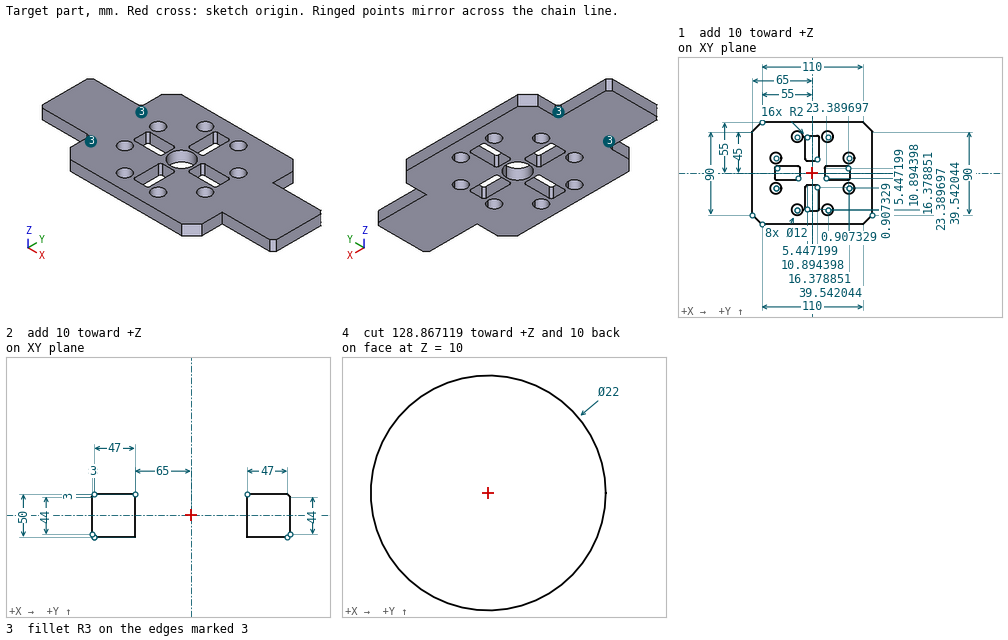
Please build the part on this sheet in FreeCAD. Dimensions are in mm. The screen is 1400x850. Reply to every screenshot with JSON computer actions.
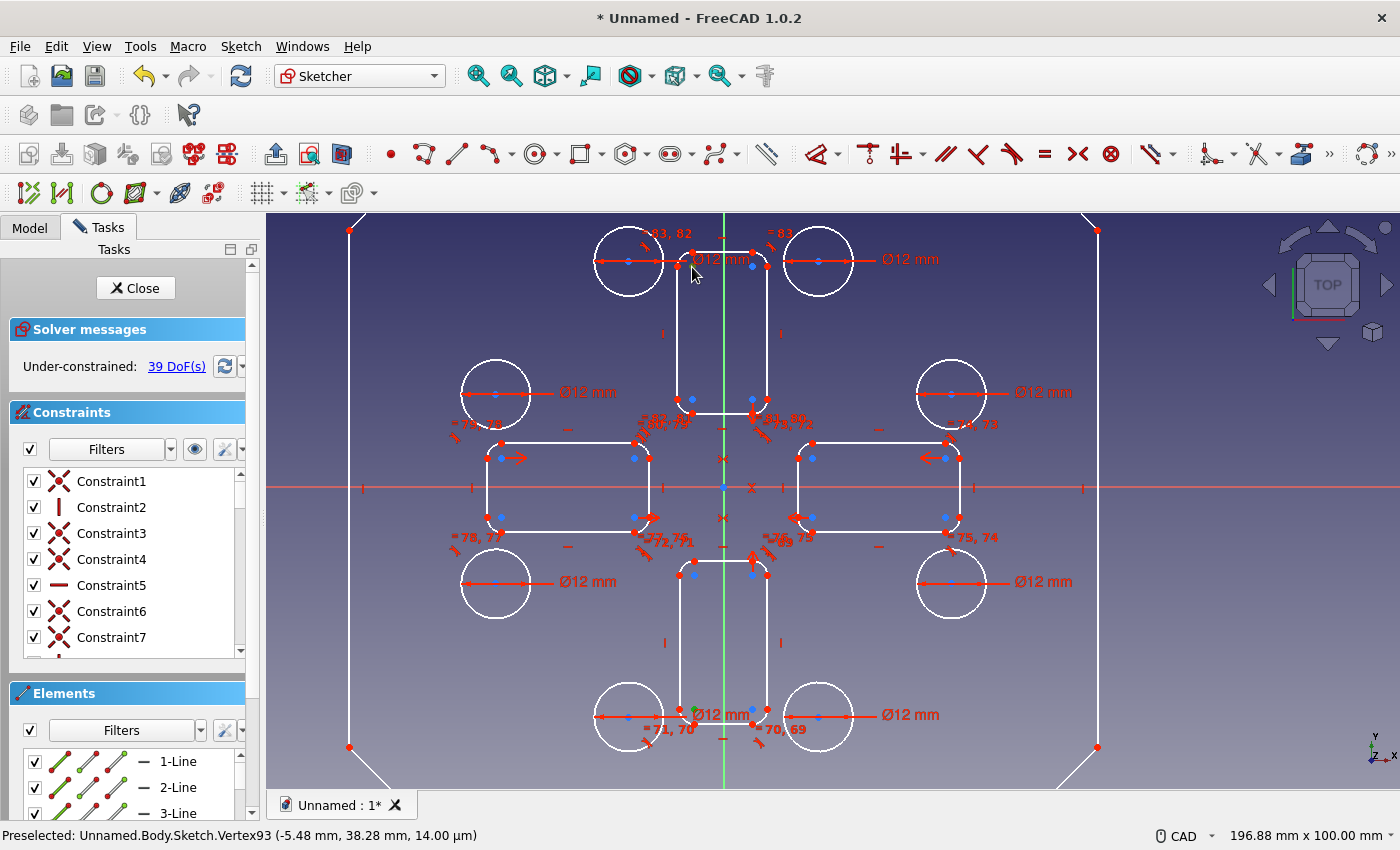
{"action": "left_click", "coordinate": [428, 487]}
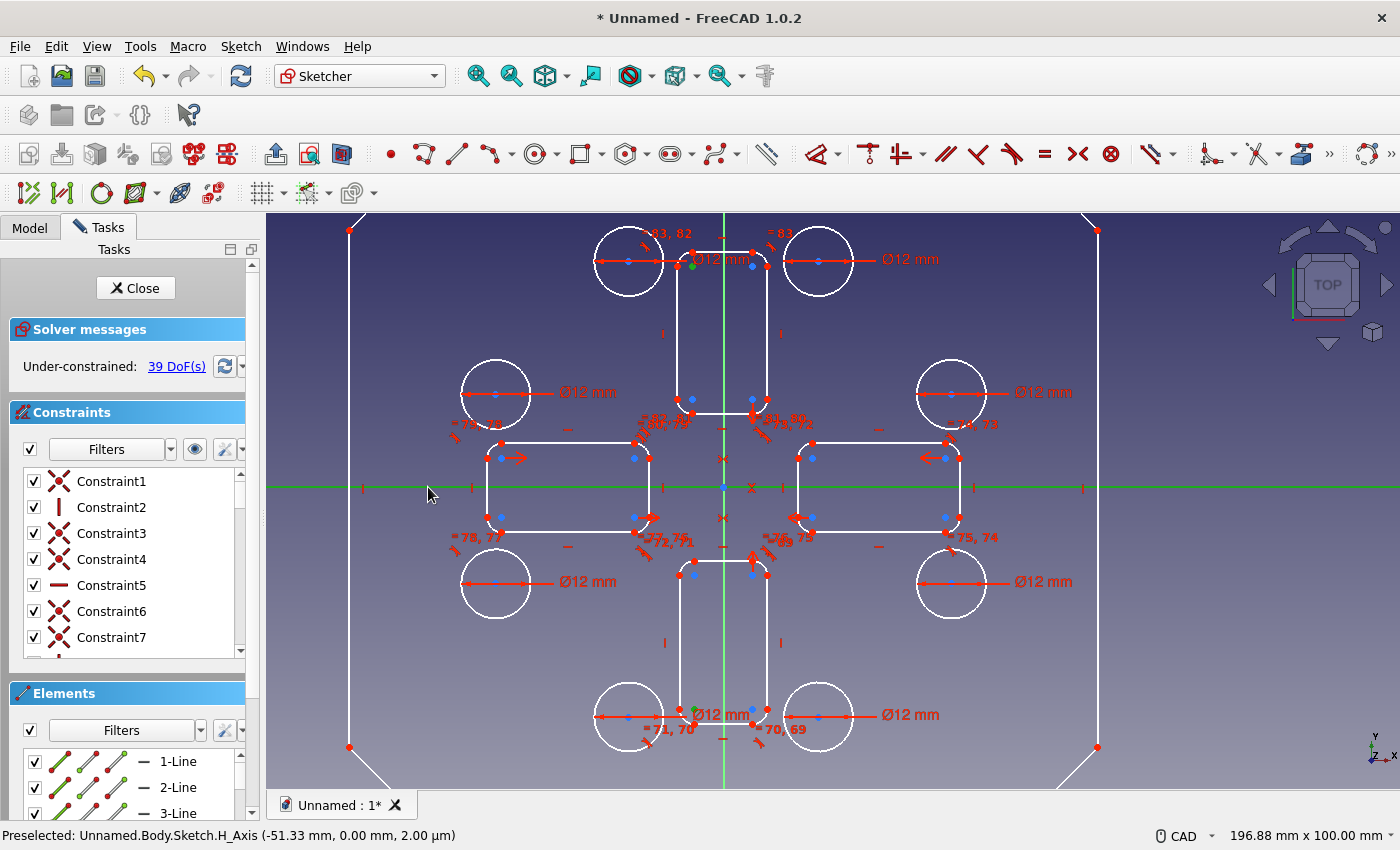
{"action": "left_click", "coordinate": [1078, 154]}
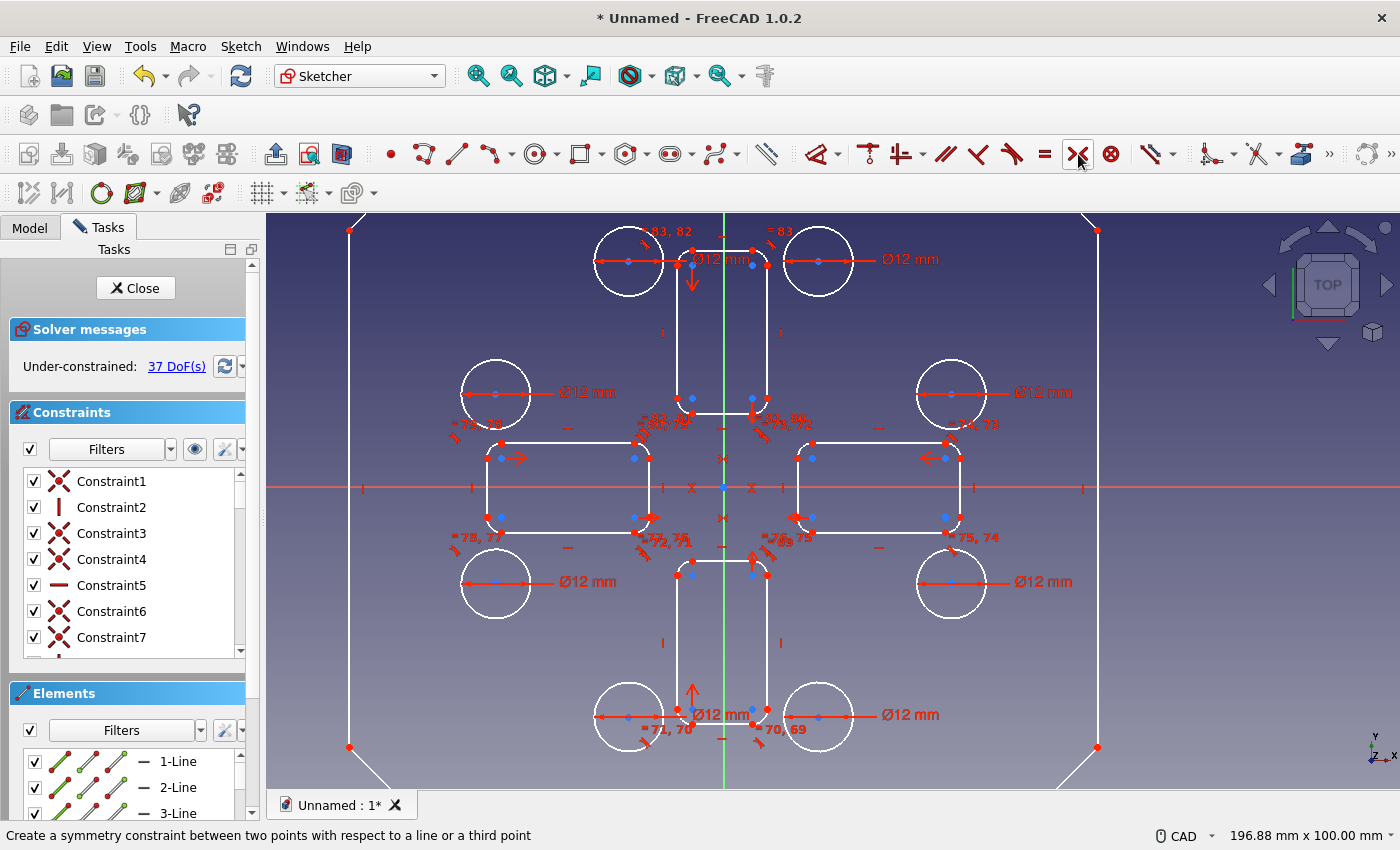
{"action": "left_click", "coordinate": [818, 717]}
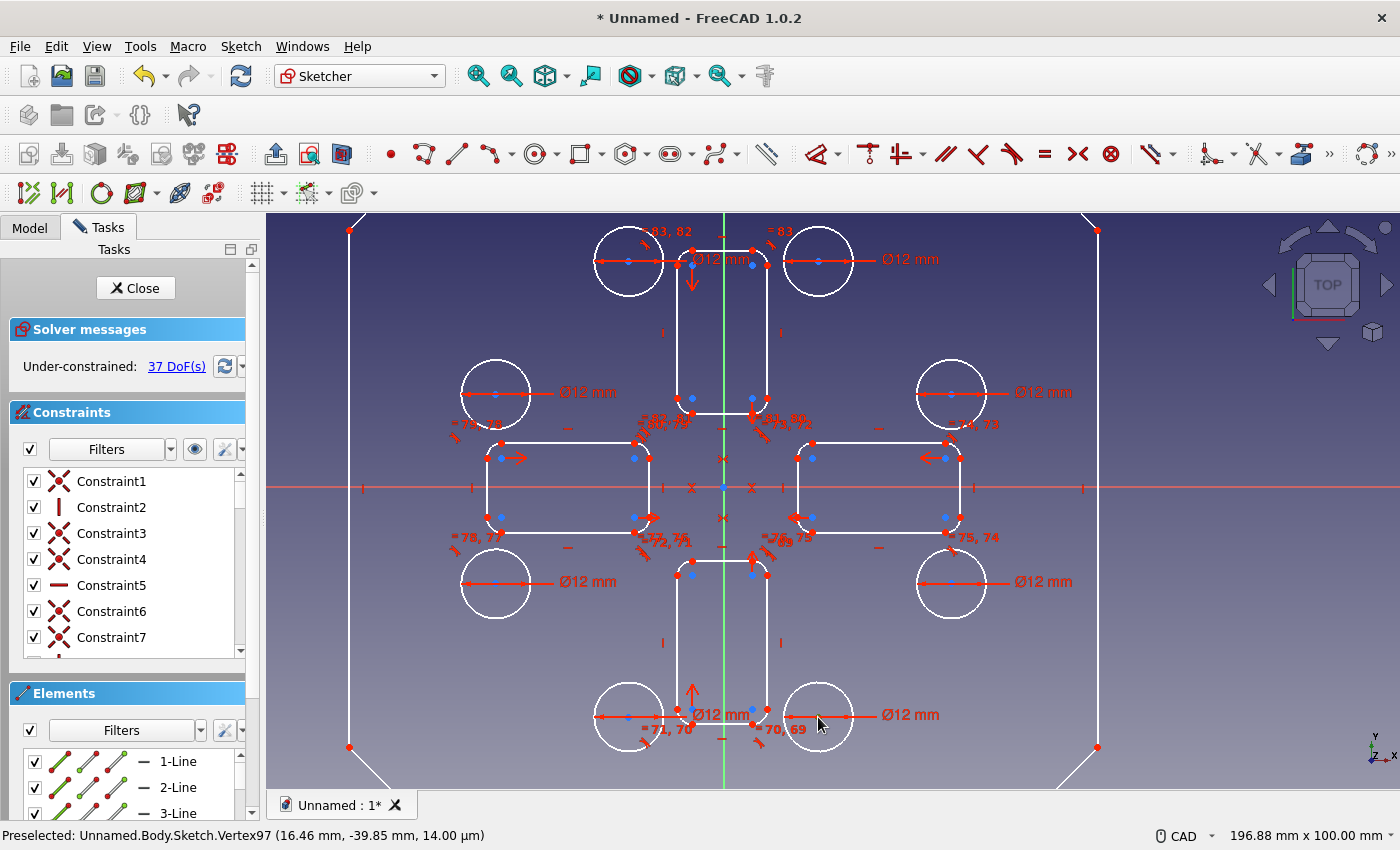
{"action": "left_click", "coordinate": [629, 717]}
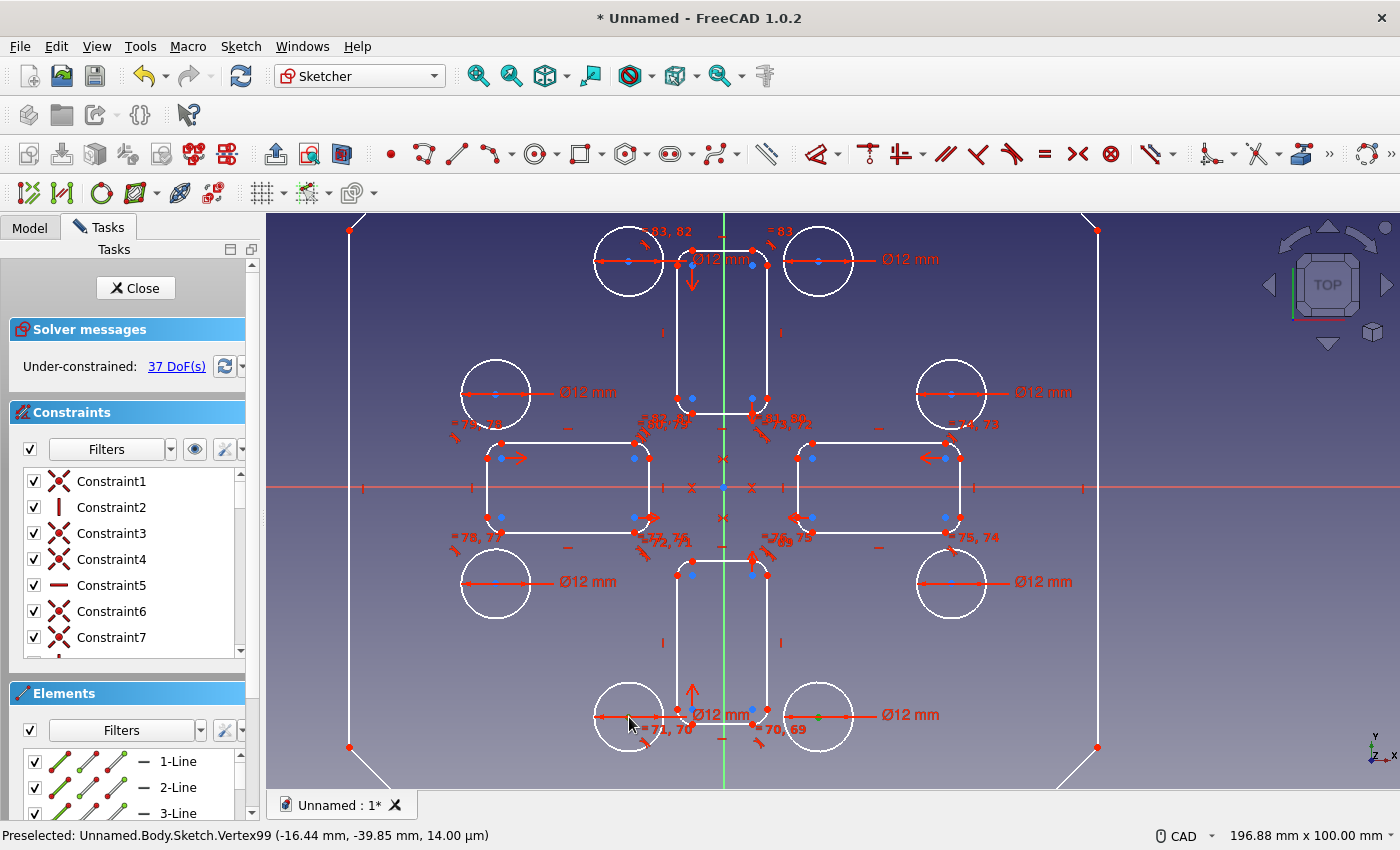
{"action": "left_click", "coordinate": [724, 687]}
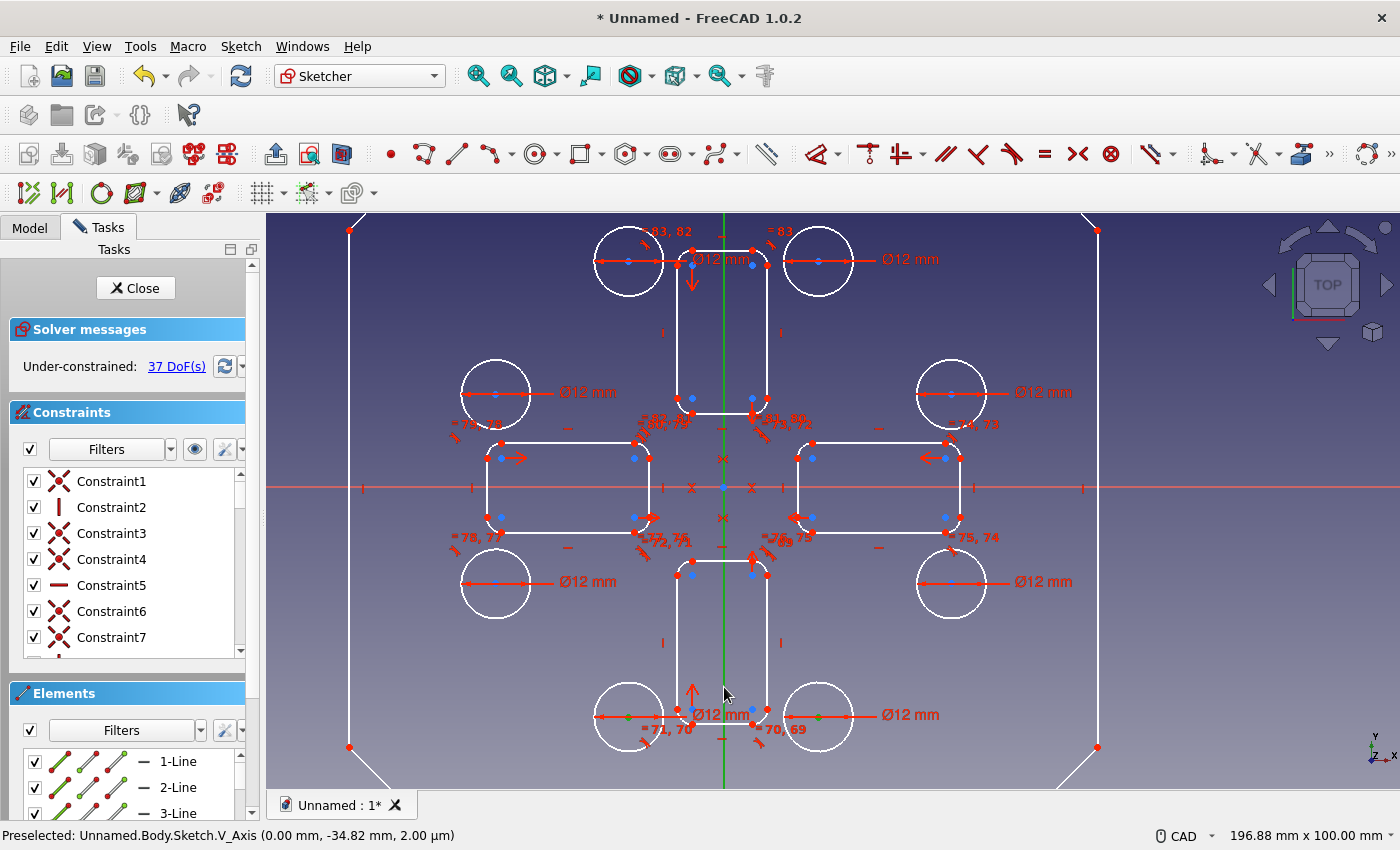
{"action": "left_click", "coordinate": [1078, 154]}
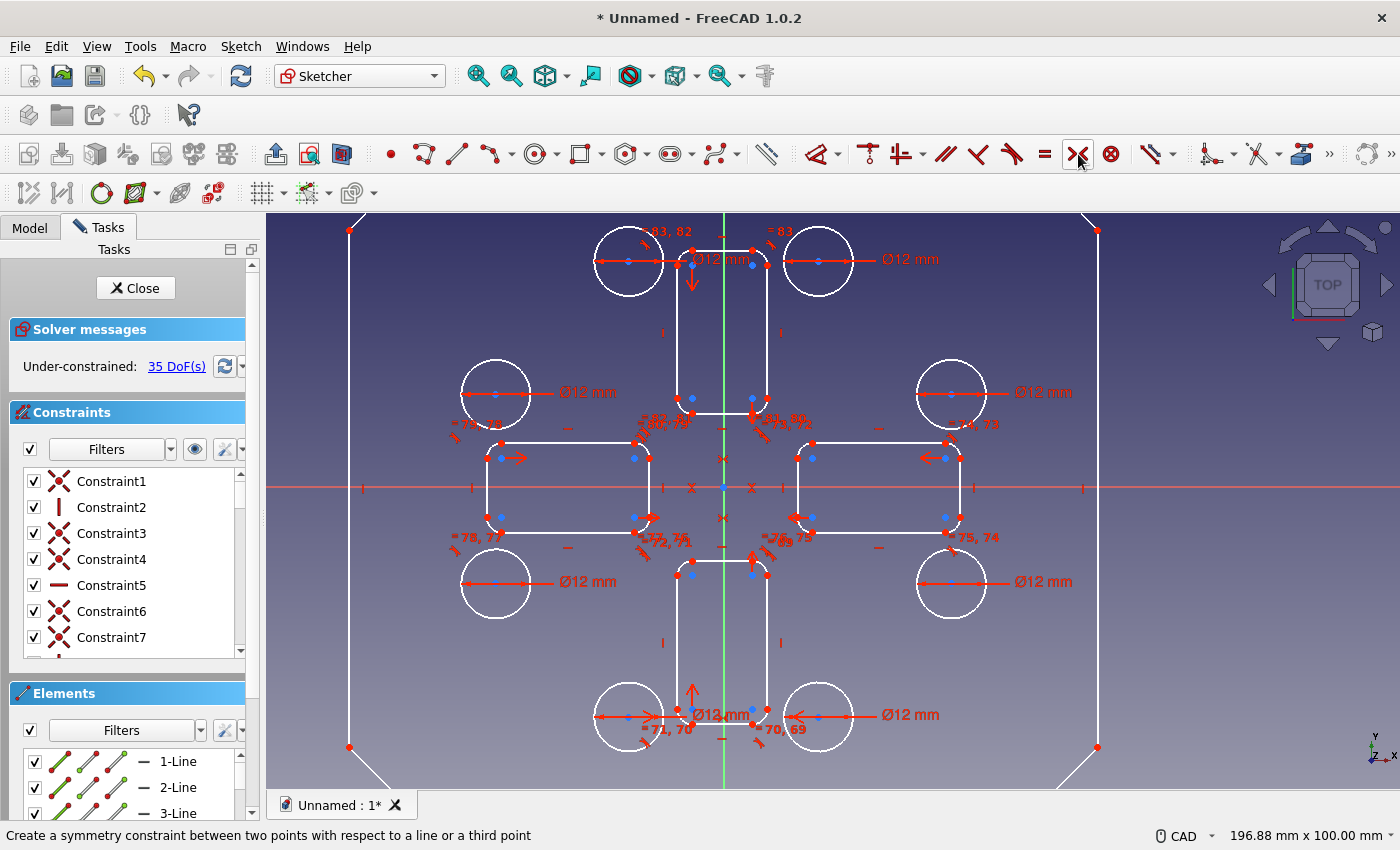
{"action": "left_click", "coordinate": [951, 584]}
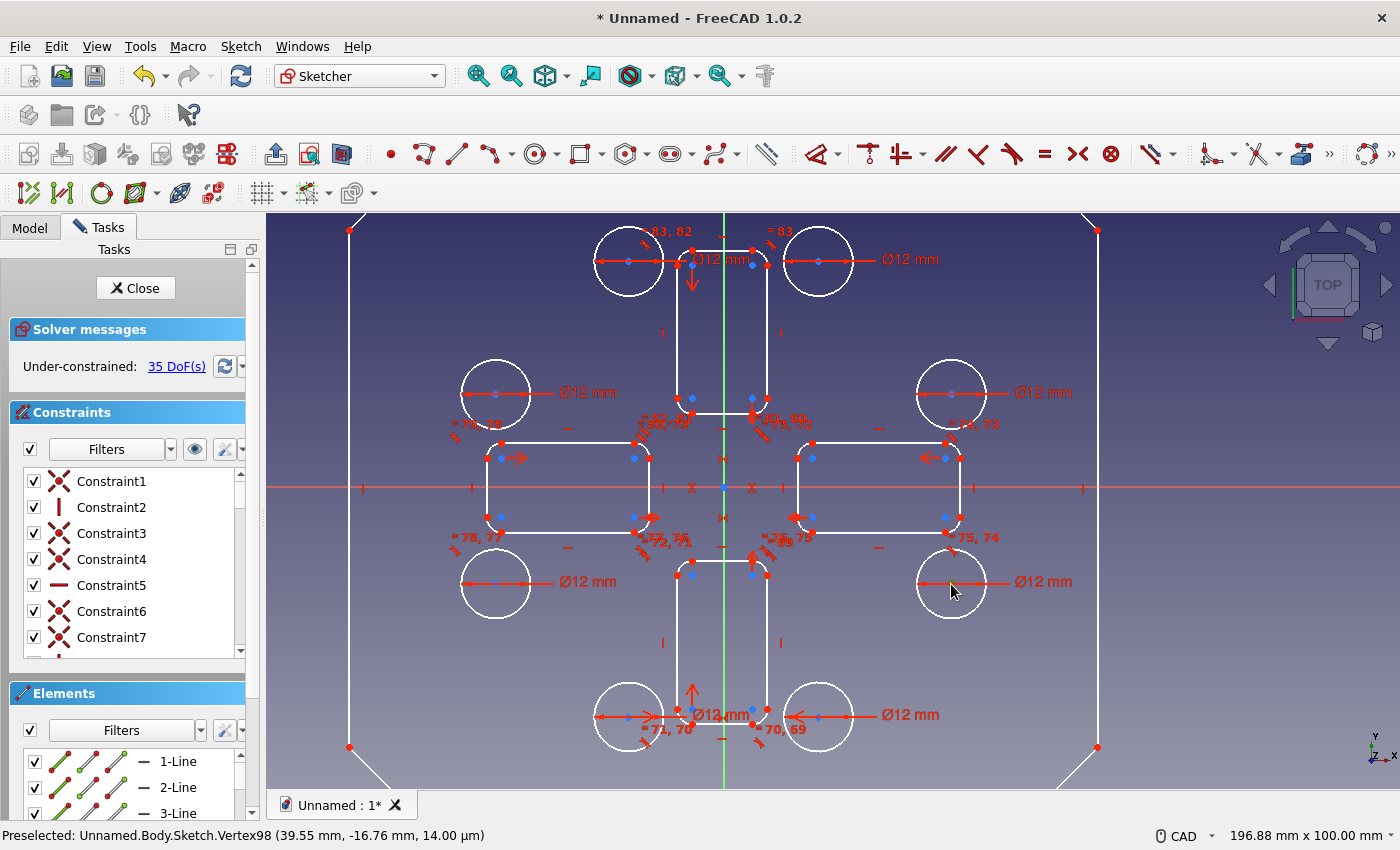
{"action": "left_click", "coordinate": [496, 584]}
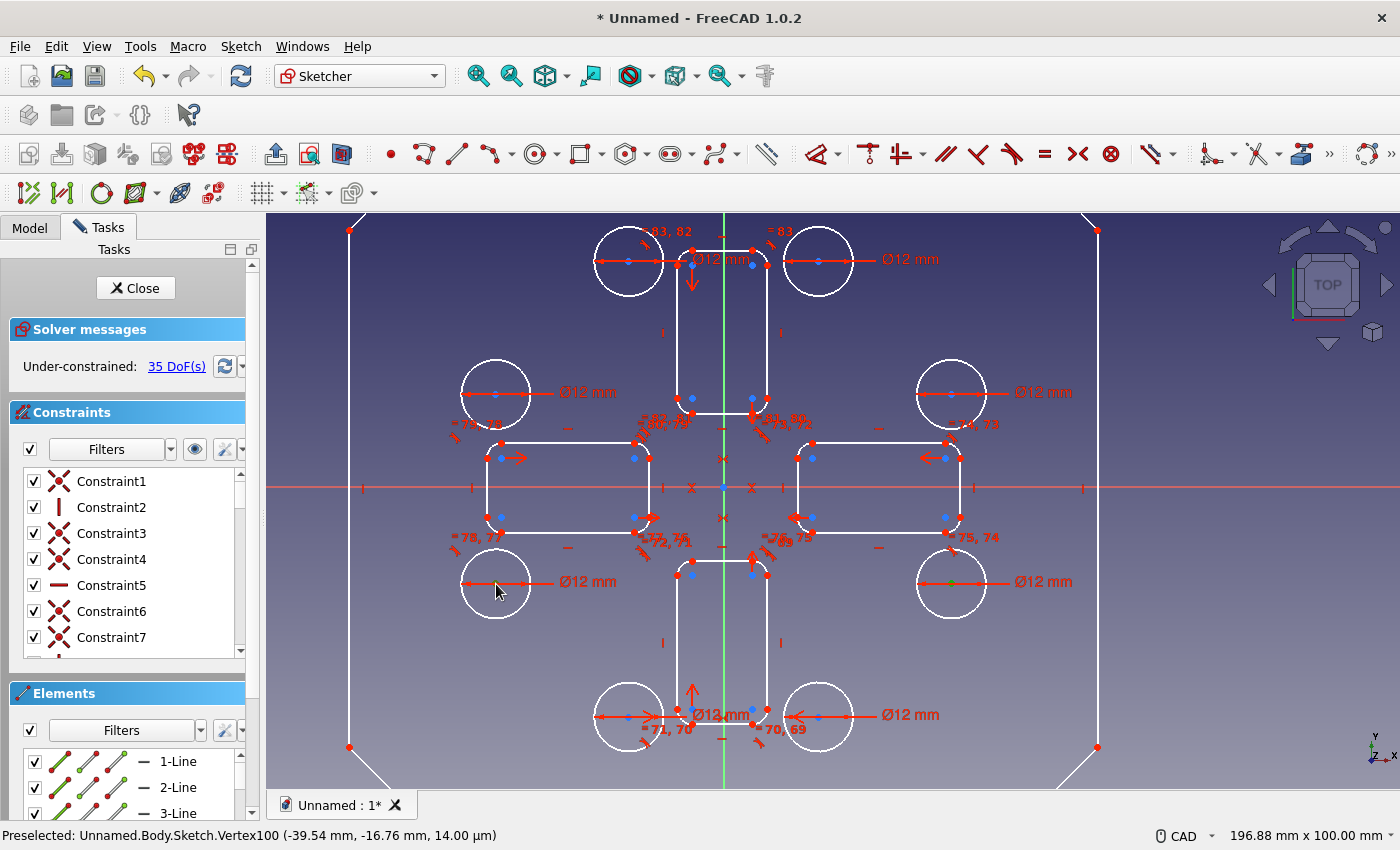
{"action": "left_click", "coordinate": [724, 687]}